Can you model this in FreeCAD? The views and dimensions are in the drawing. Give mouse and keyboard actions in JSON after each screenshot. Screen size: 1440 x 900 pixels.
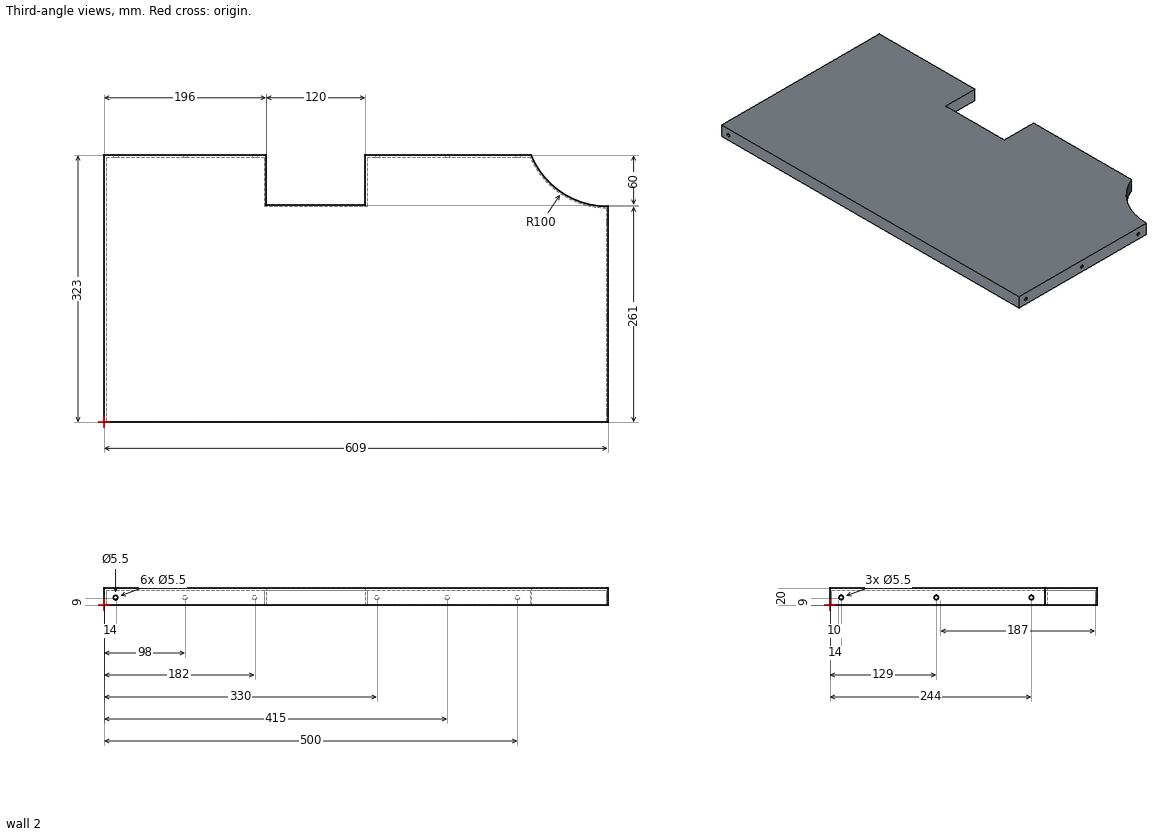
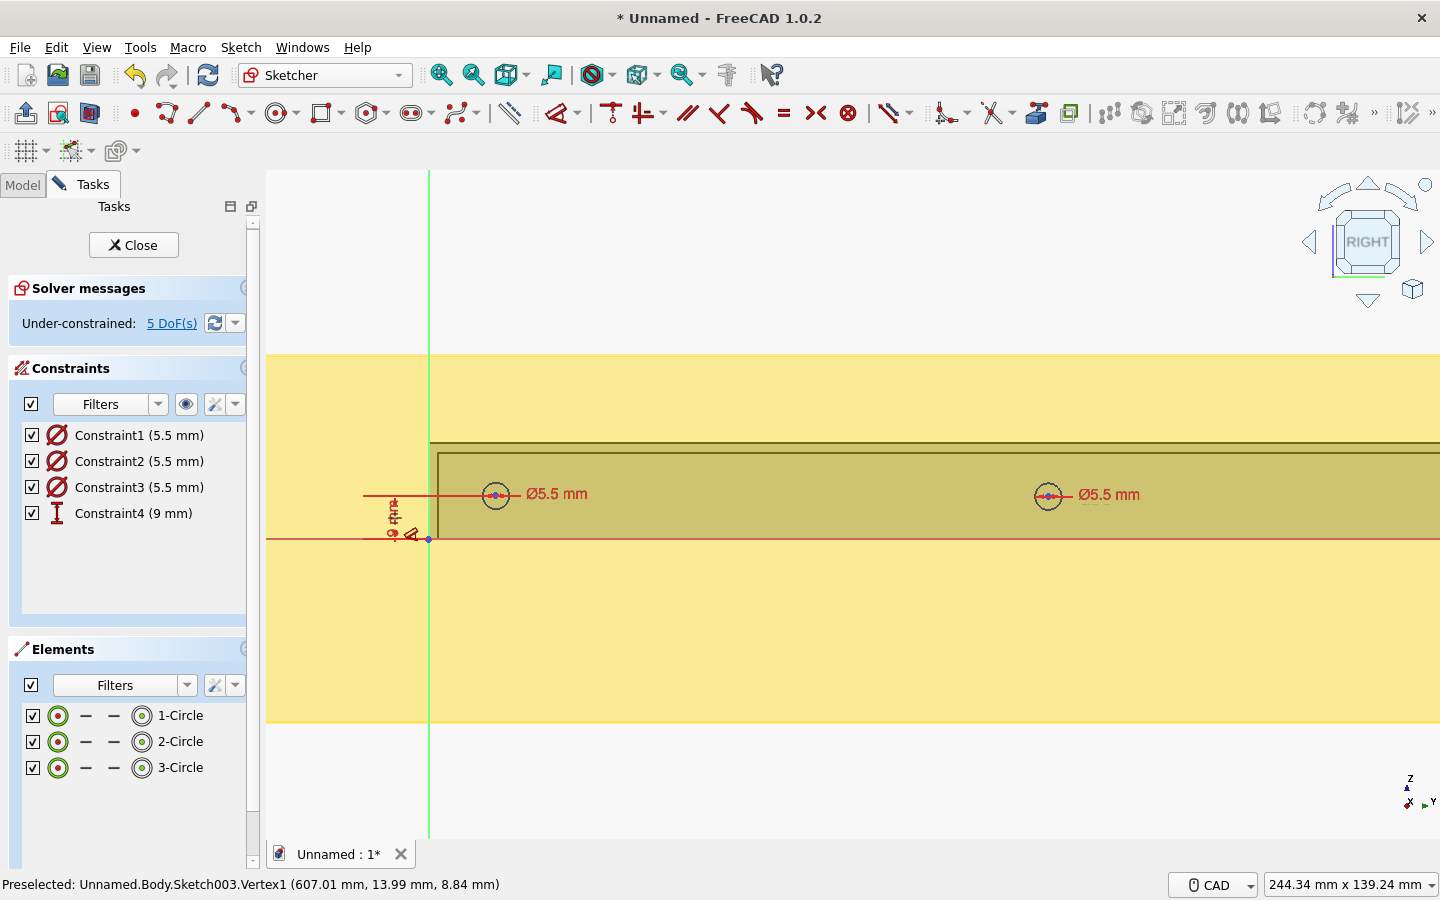
{"action": "left_click", "coordinate": [1048, 497]}
{"action": "left_click", "coordinate": [1082, 518]}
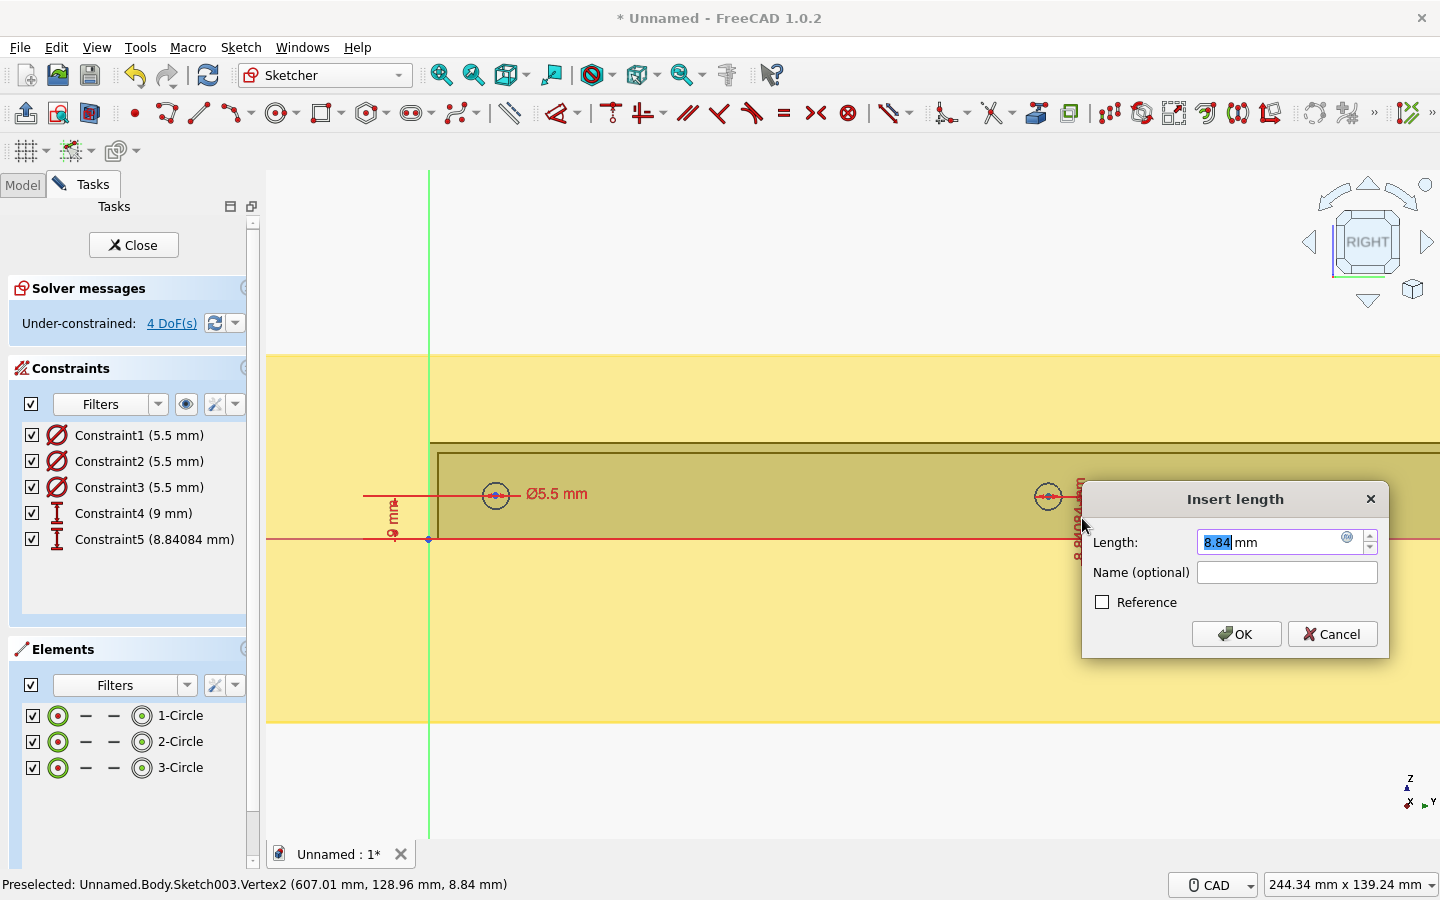
{"action": "type", "text": "9"}
{"action": "key", "text": "Return"}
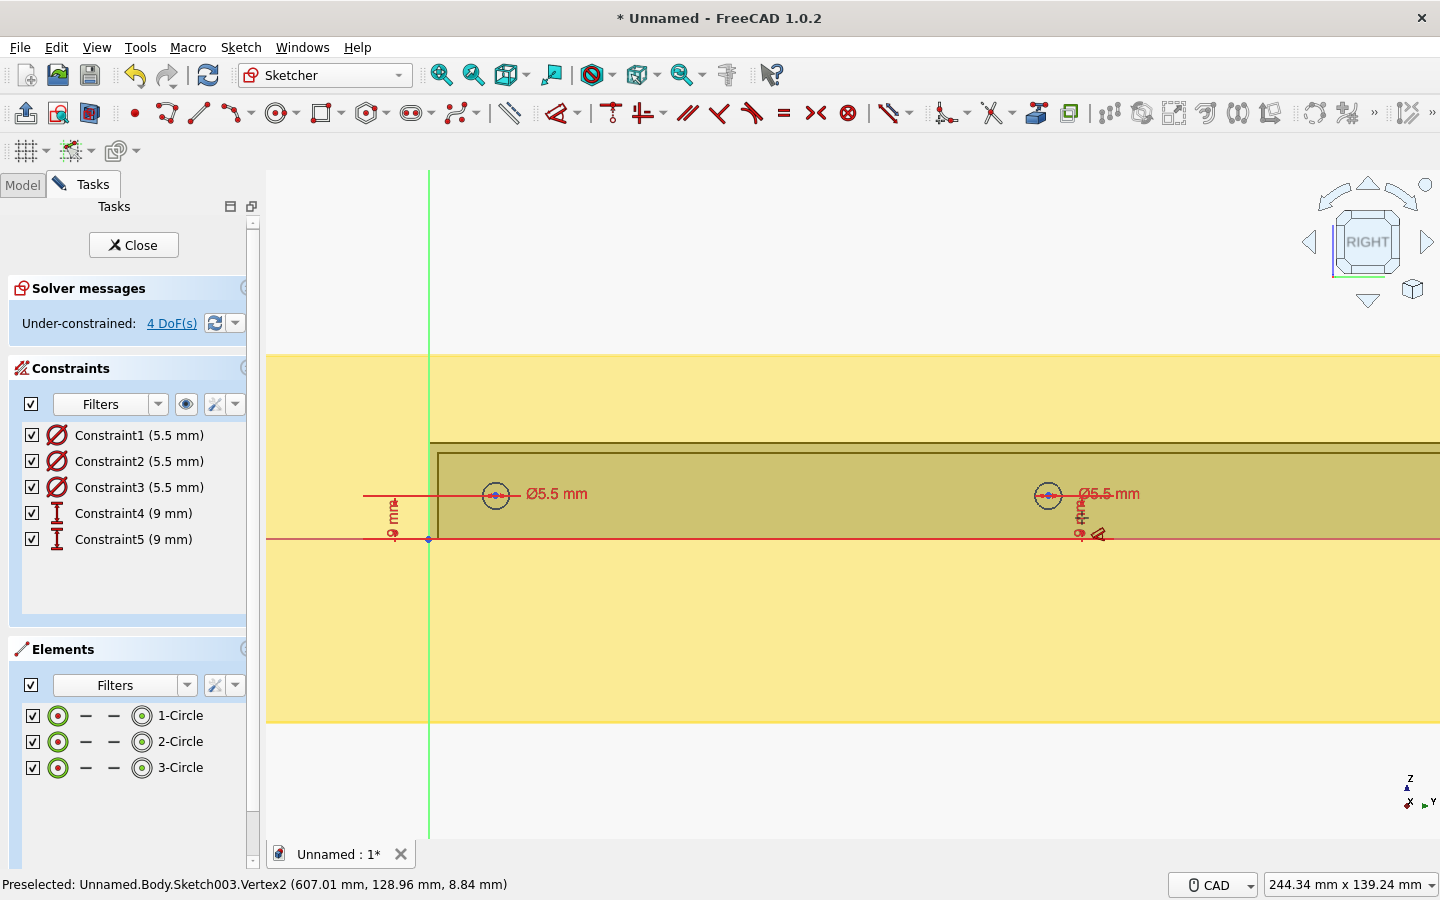
{"action": "scroll", "coordinate": [496, 497], "scroll_direction": "down", "scroll_amount": 3}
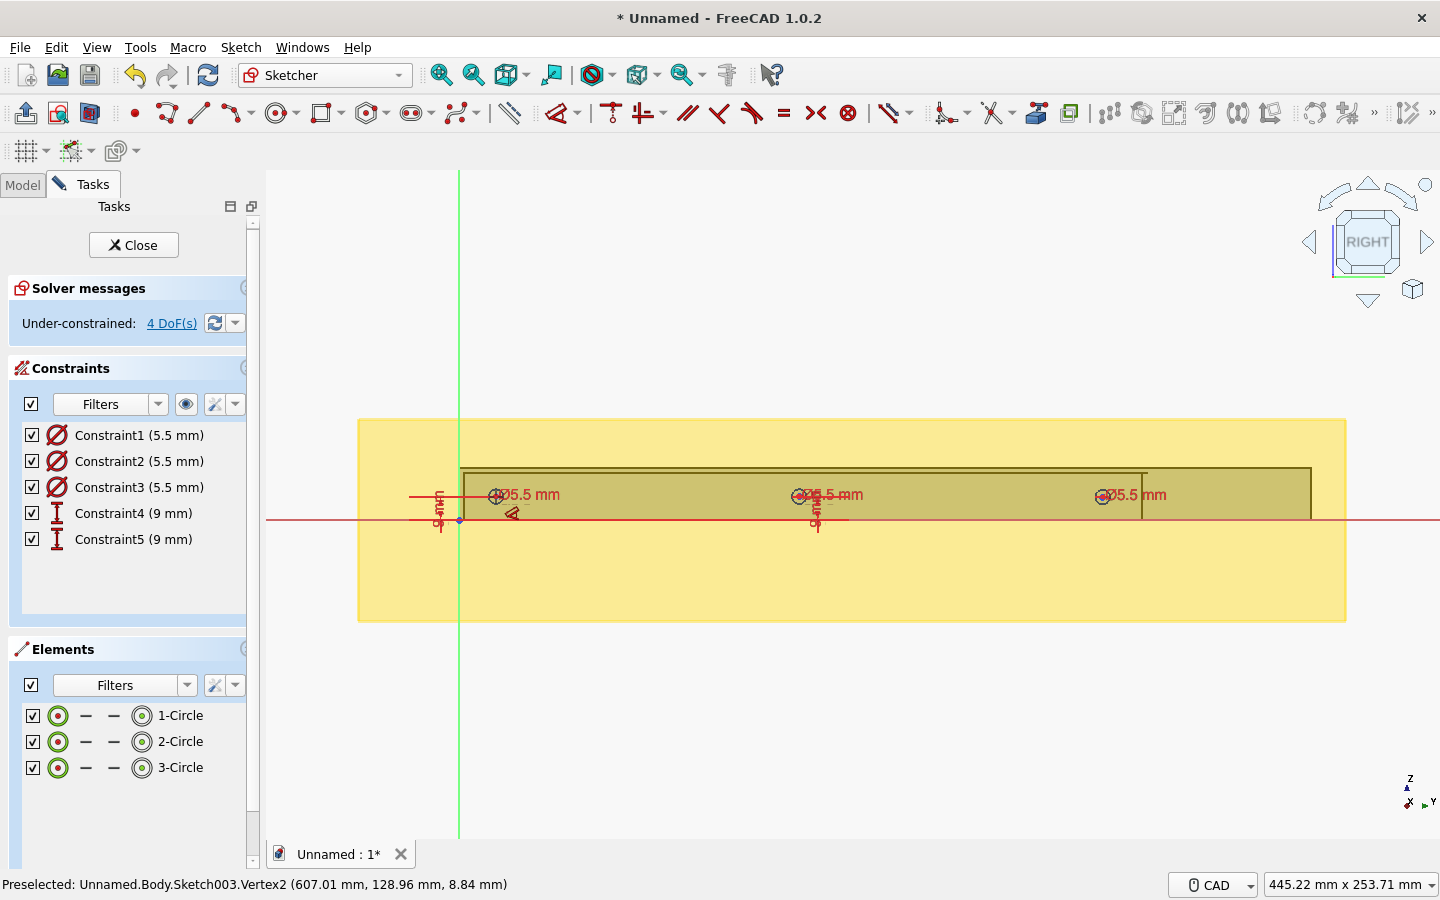
{"action": "scroll", "coordinate": [1103, 497], "scroll_direction": "up", "scroll_amount": 3}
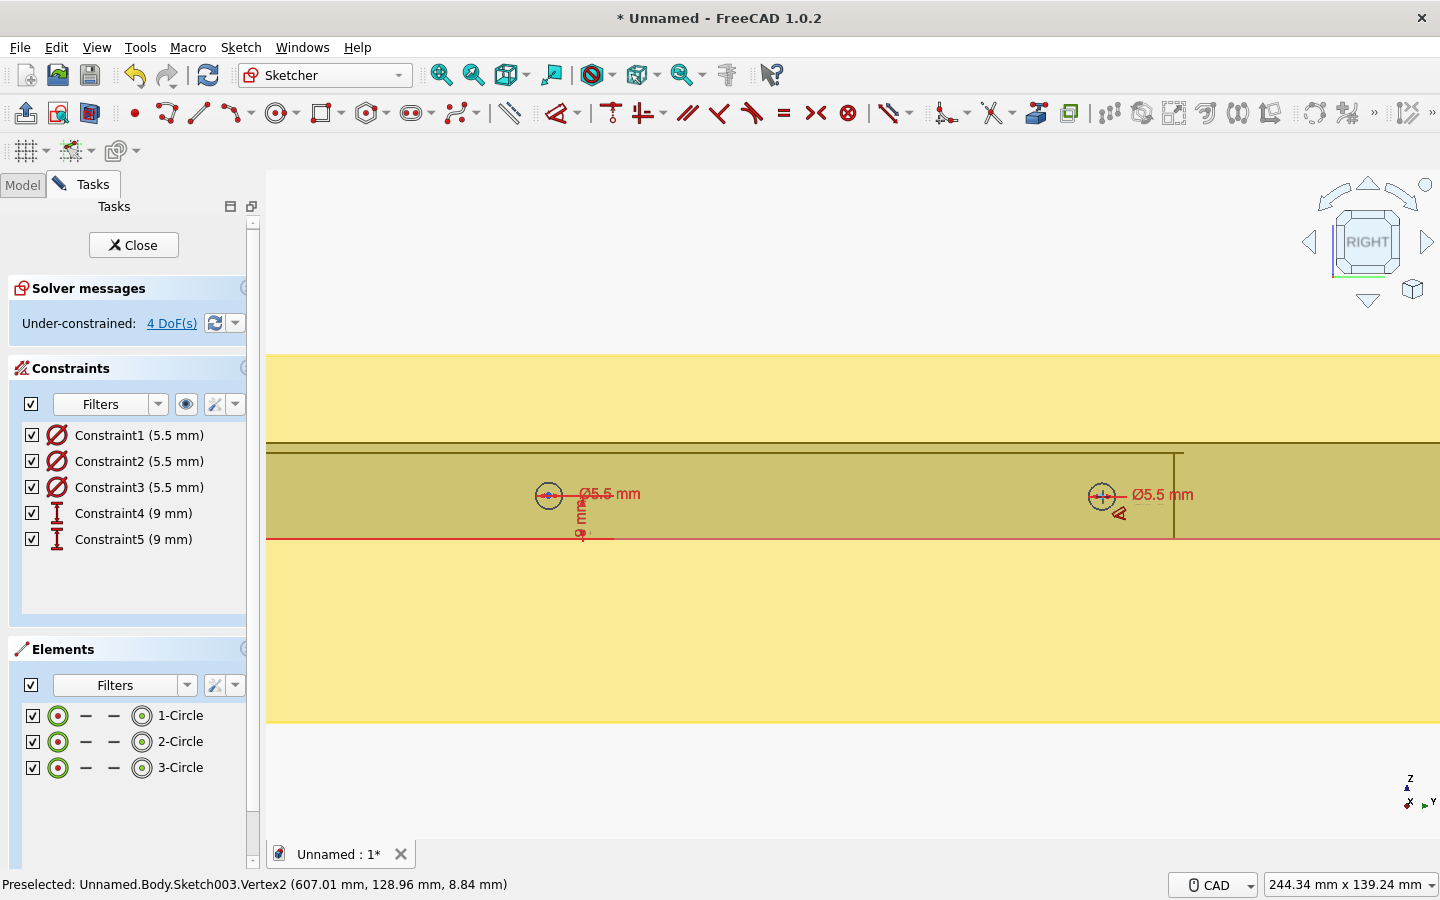
{"action": "left_click", "coordinate": [1102, 497]}
{"action": "left_click", "coordinate": [1136, 518]}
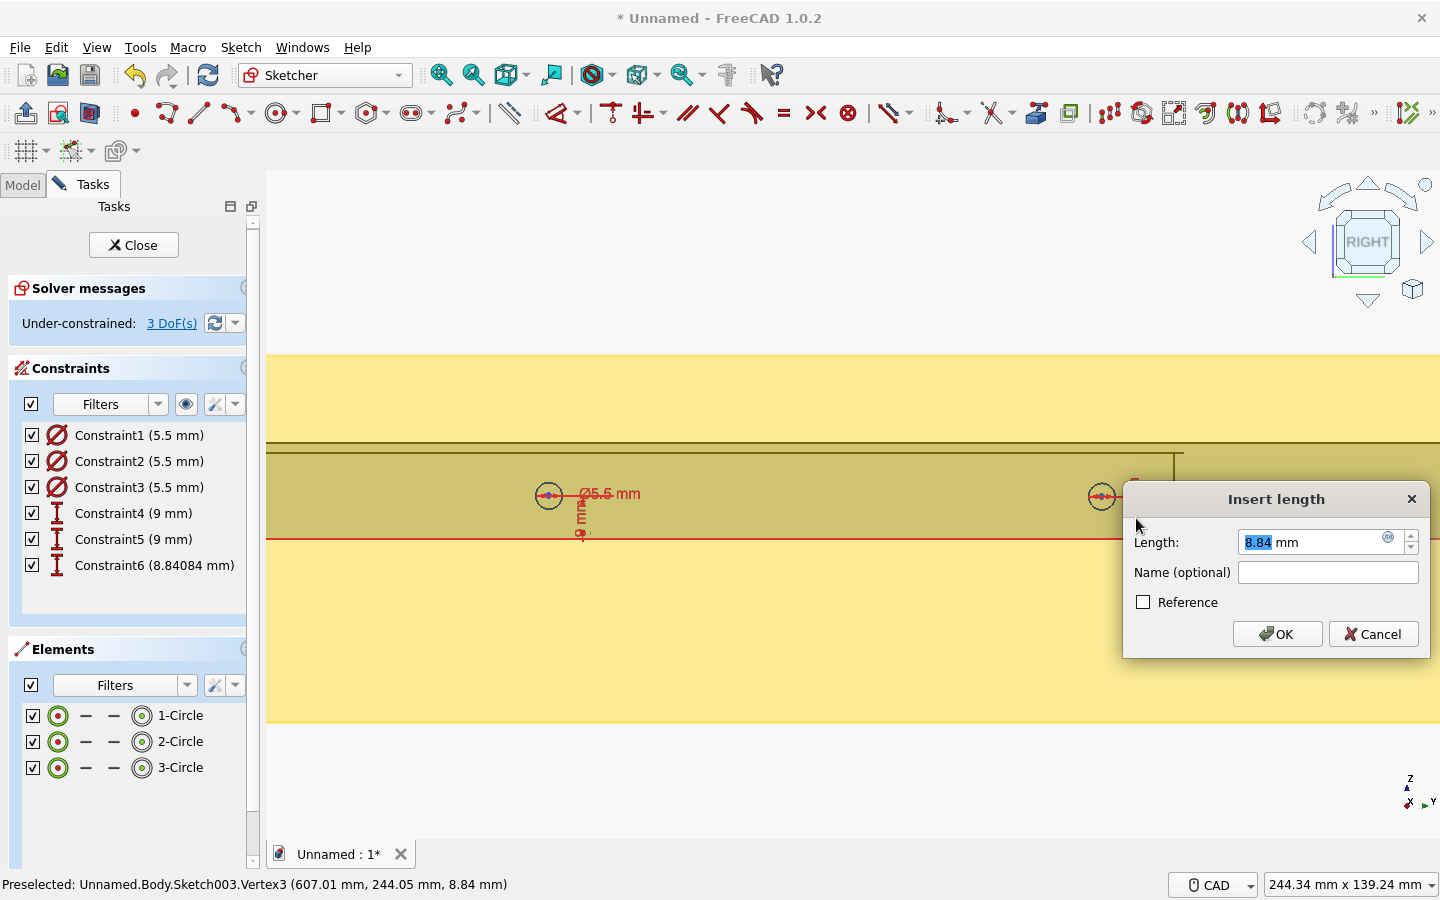
{"action": "type", "text": "9"}
{"action": "key", "text": "Return"}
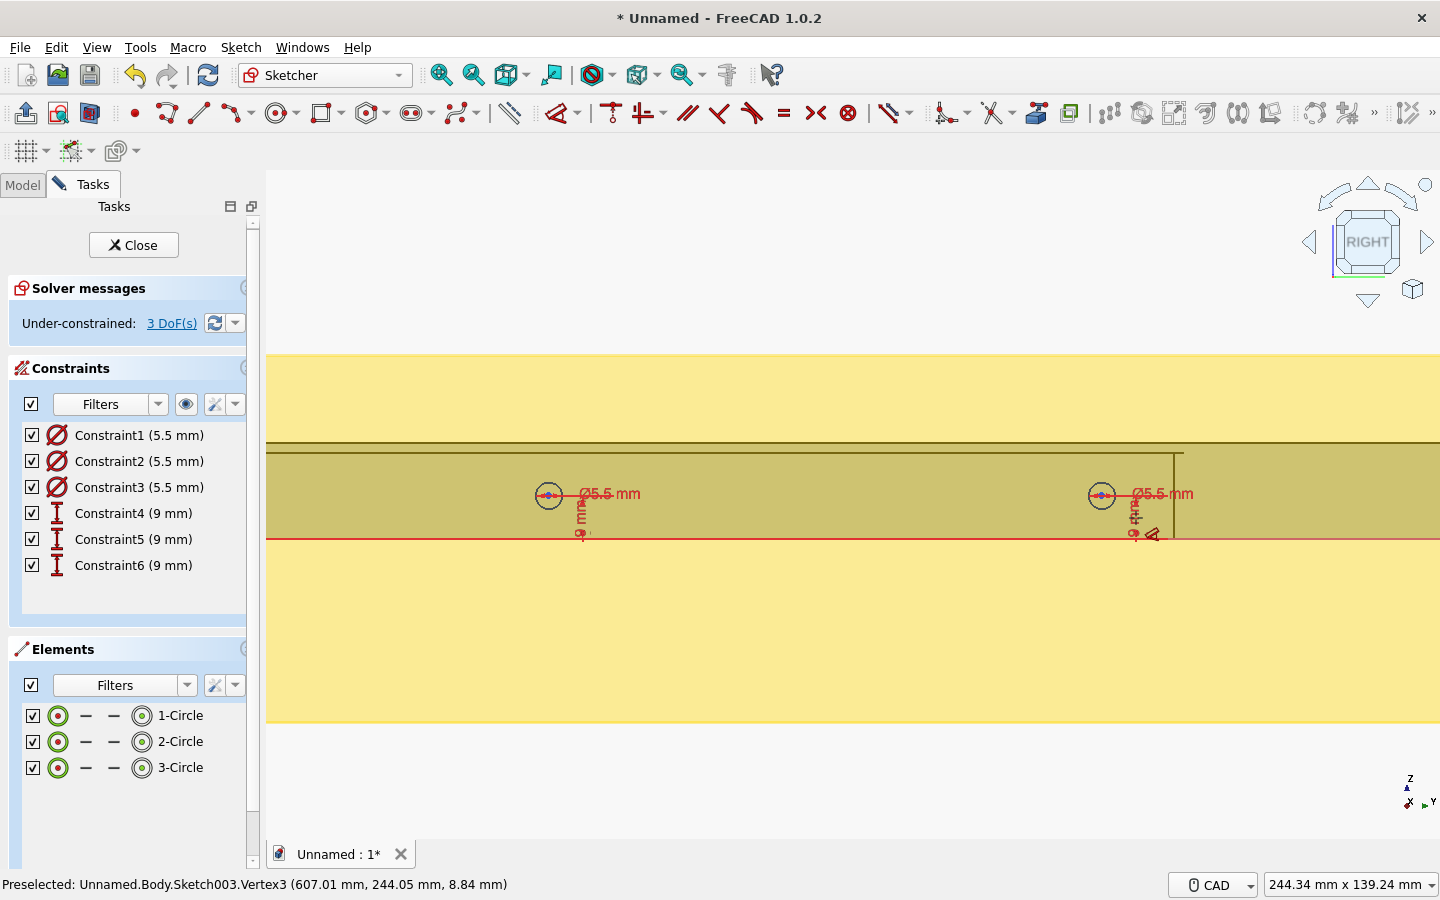
{"action": "scroll", "coordinate": [1104, 497], "scroll_direction": "down", "scroll_amount": 3}